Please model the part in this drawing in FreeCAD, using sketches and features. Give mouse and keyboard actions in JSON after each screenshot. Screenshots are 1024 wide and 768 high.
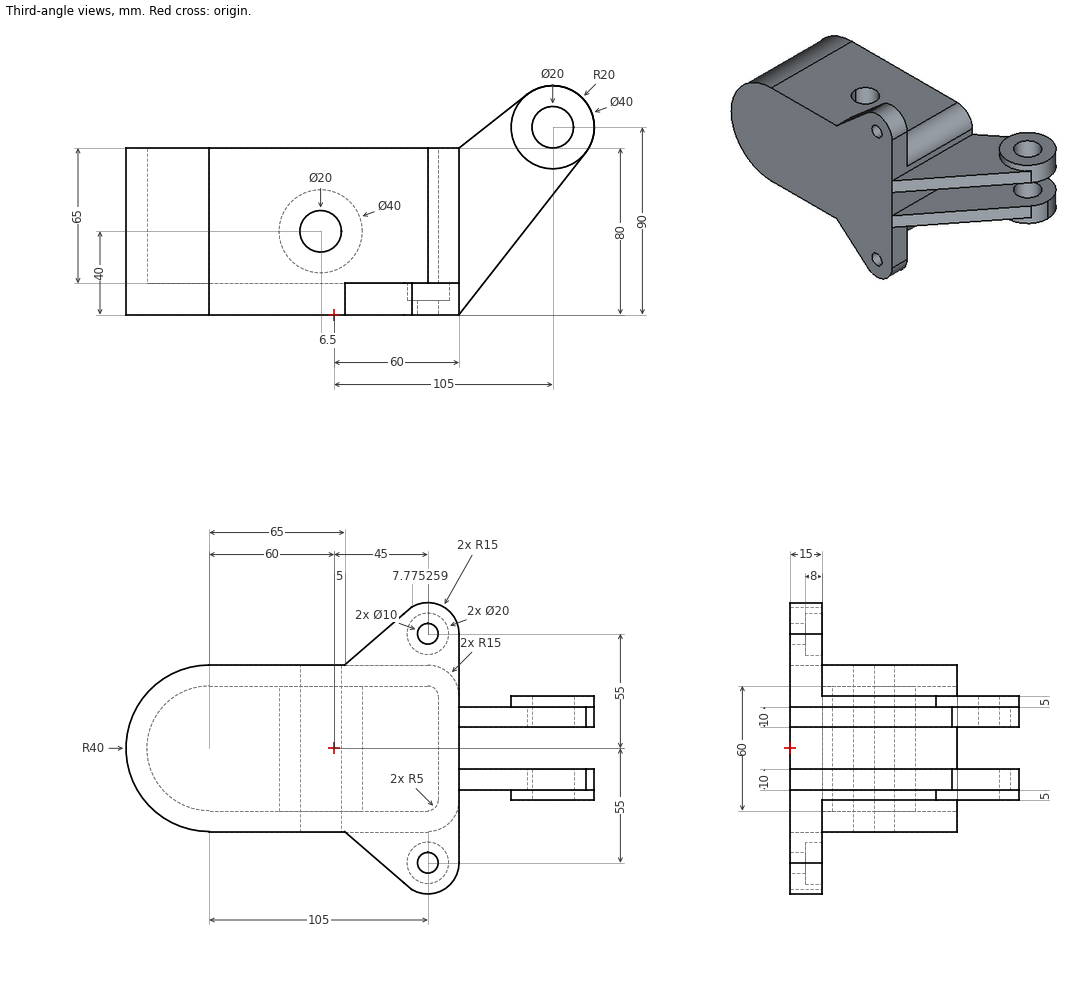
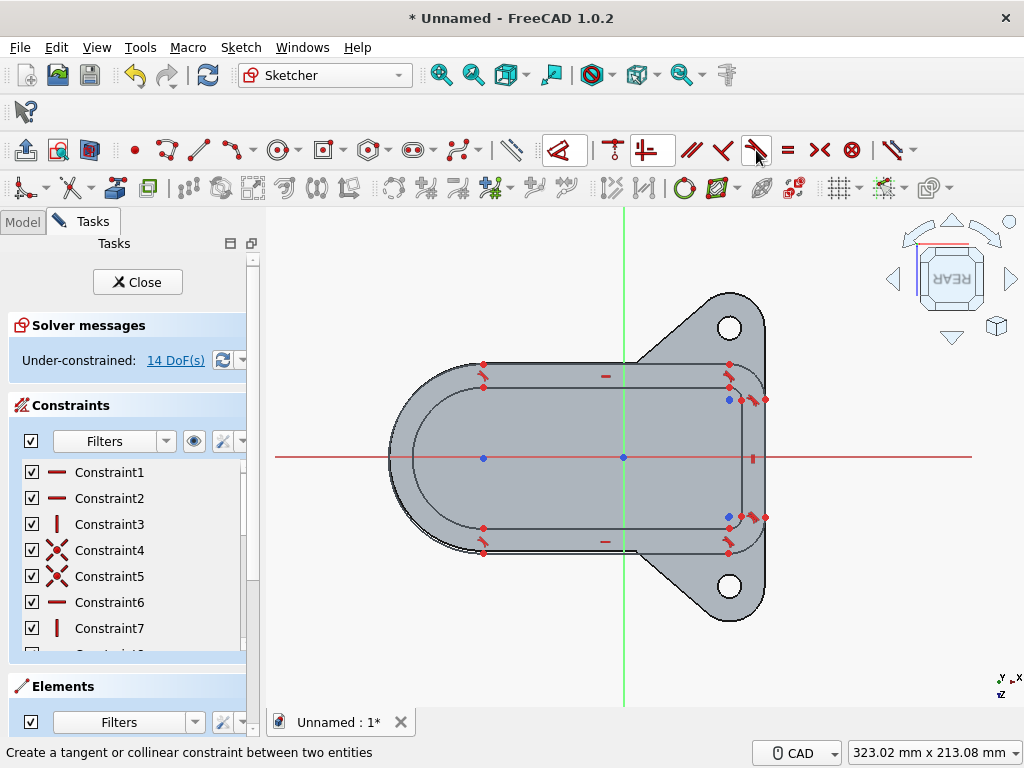
{"action": "left_click", "coordinate": [761, 384]}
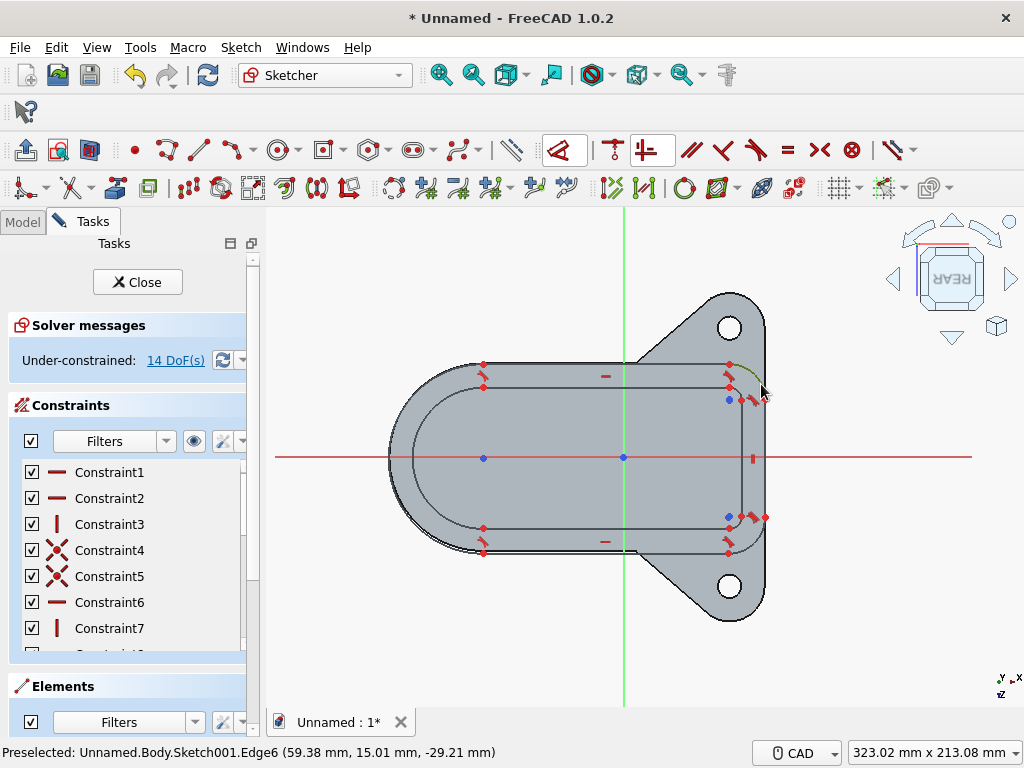
{"action": "scroll", "coordinate": [738, 391], "scroll_direction": "up", "scroll_amount": 2}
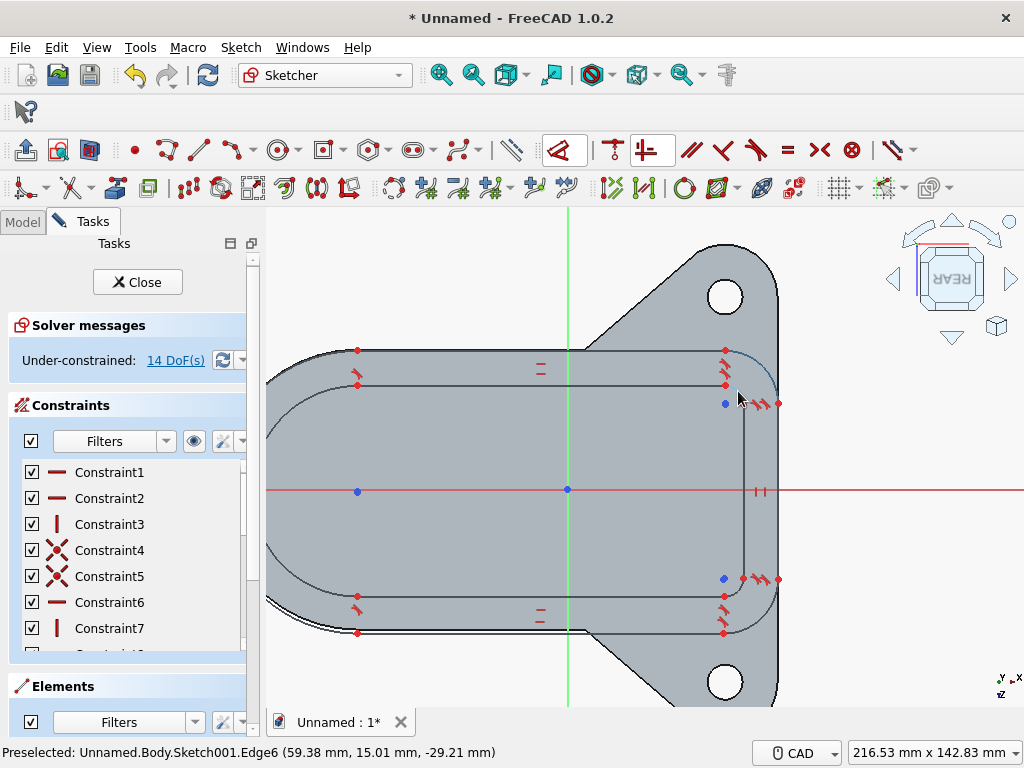
{"action": "left_click", "coordinate": [738, 391]}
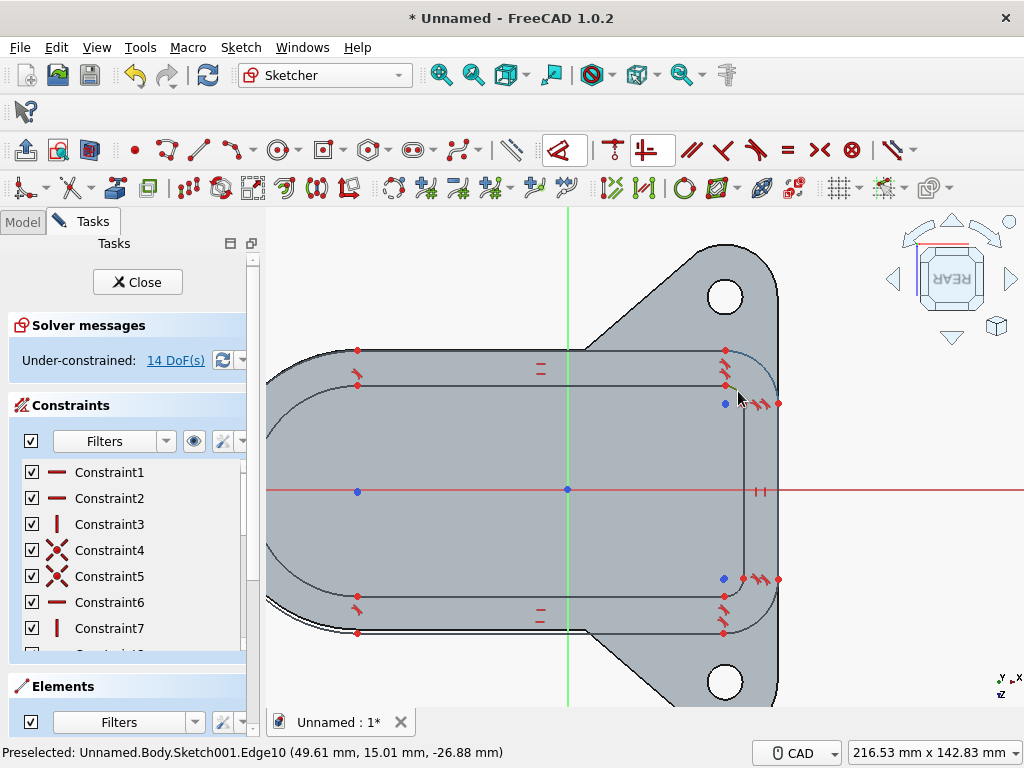
{"action": "left_click", "coordinate": [614, 150]}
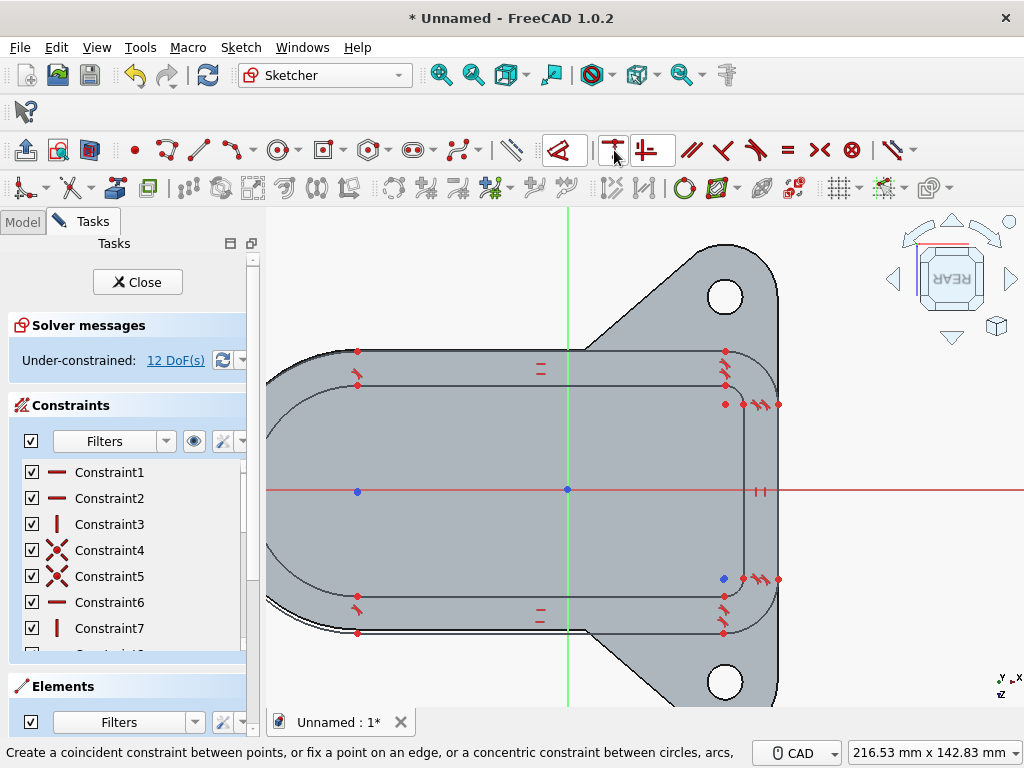
{"action": "left_click", "coordinate": [748, 628]}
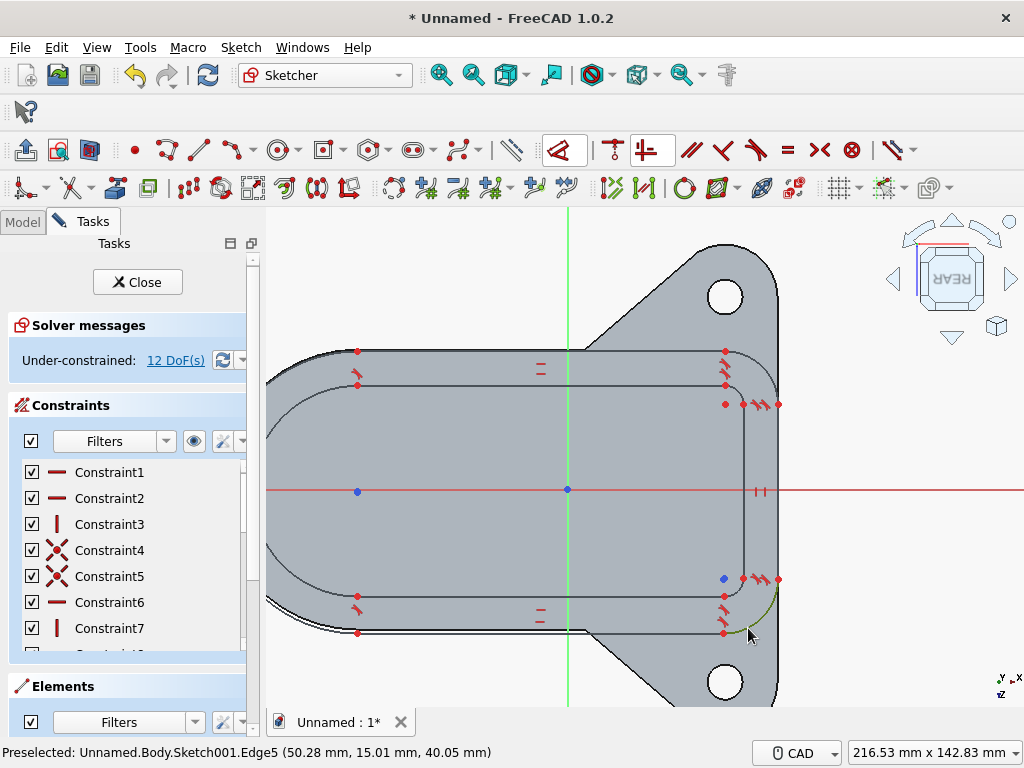
{"action": "left_click", "coordinate": [738, 591]}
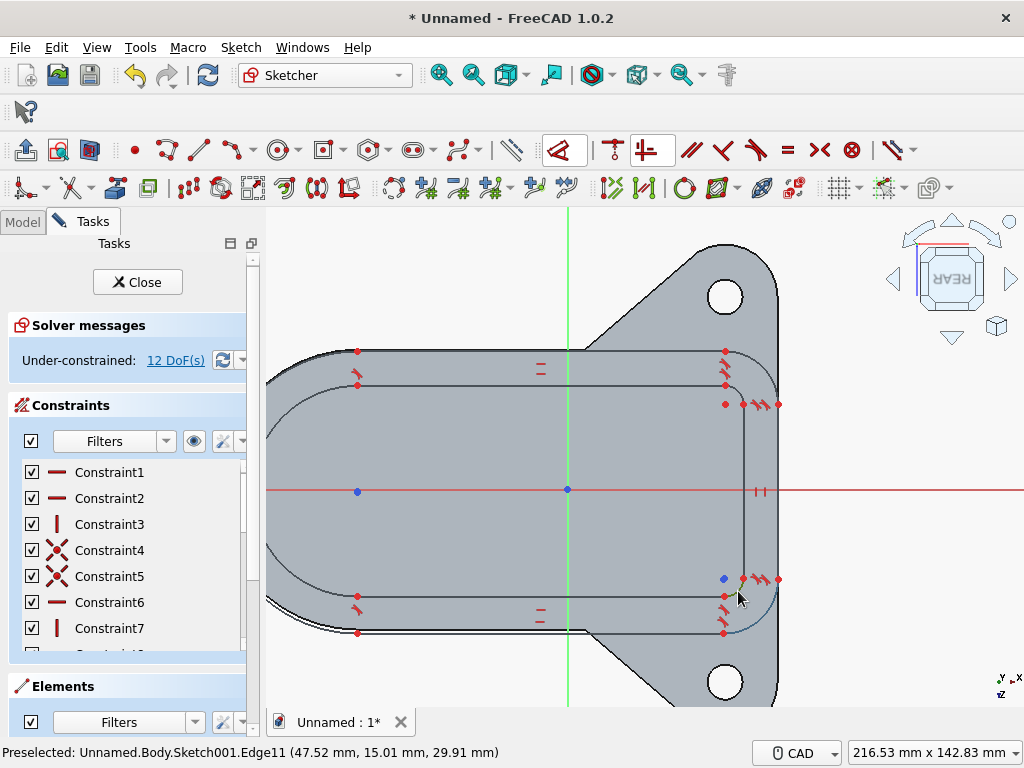
{"action": "left_click", "coordinate": [614, 150]}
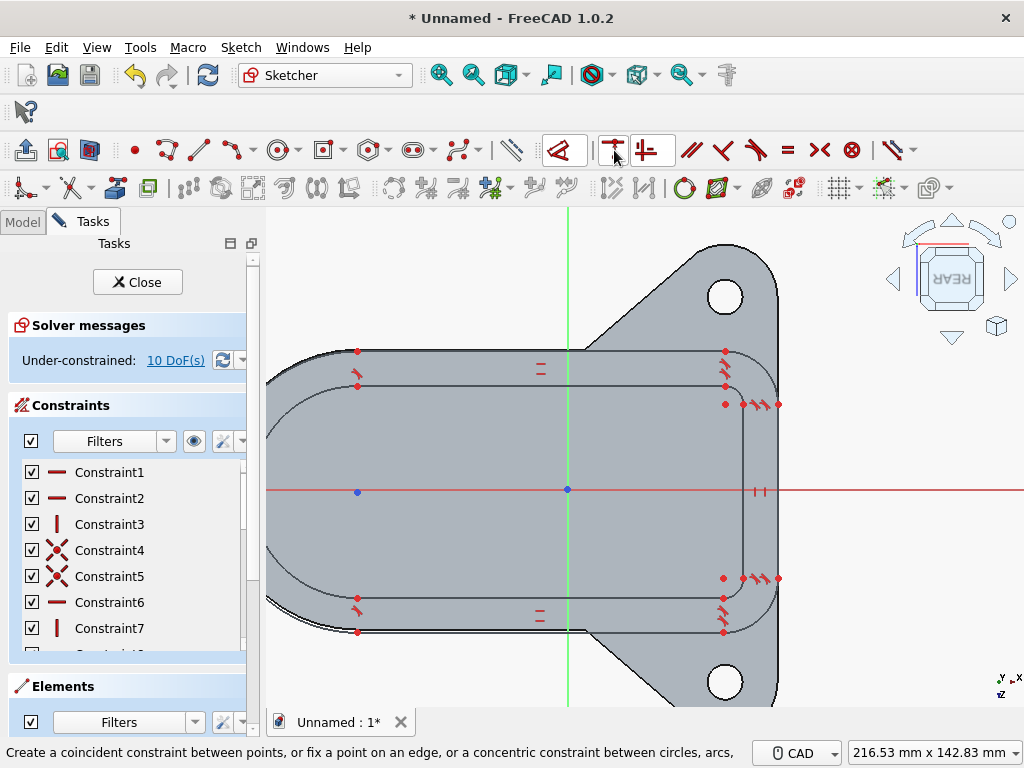
{"action": "left_click", "coordinate": [748, 627]}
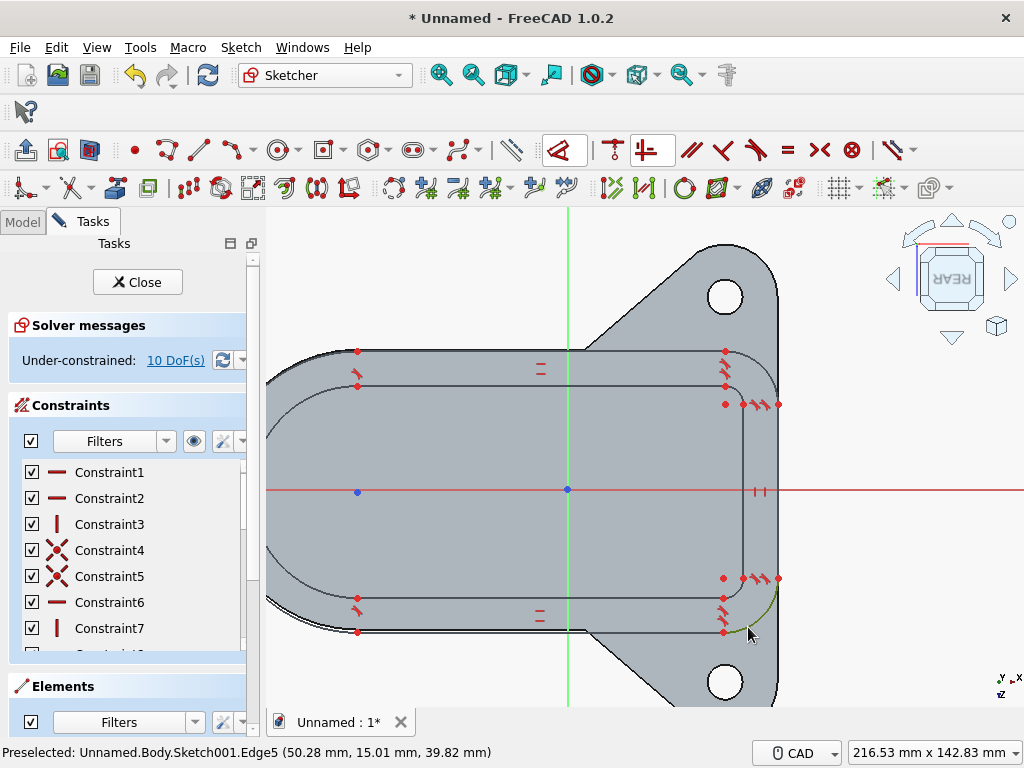
{"action": "left_click", "coordinate": [772, 380]}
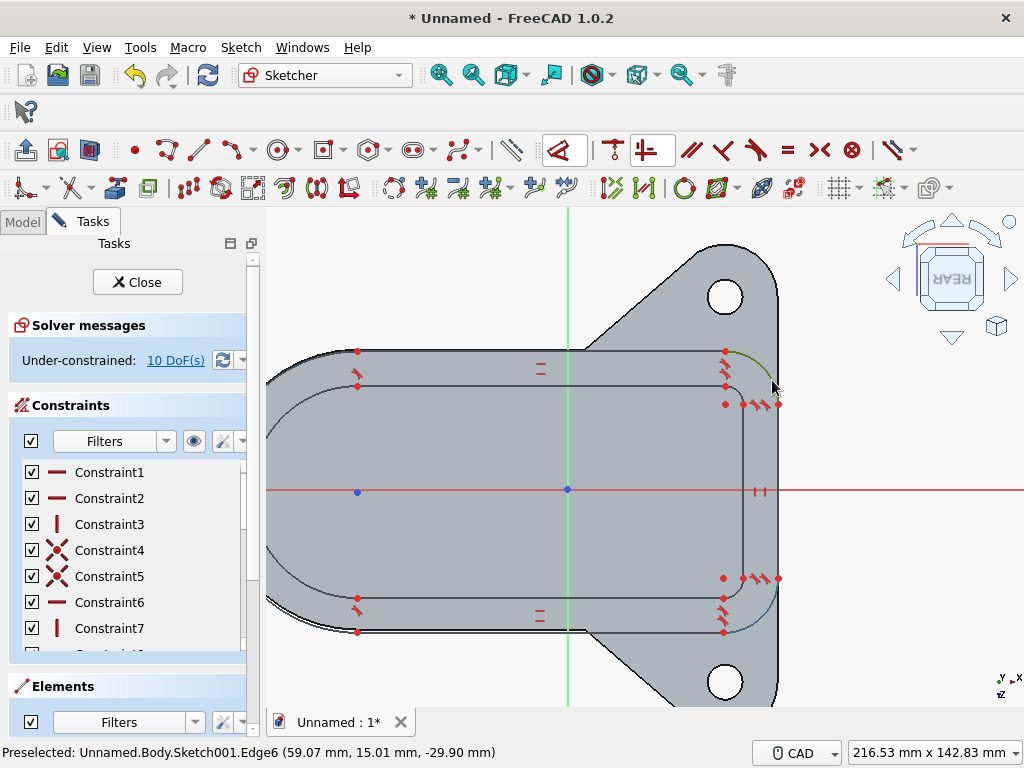
{"action": "left_click", "coordinate": [788, 150]}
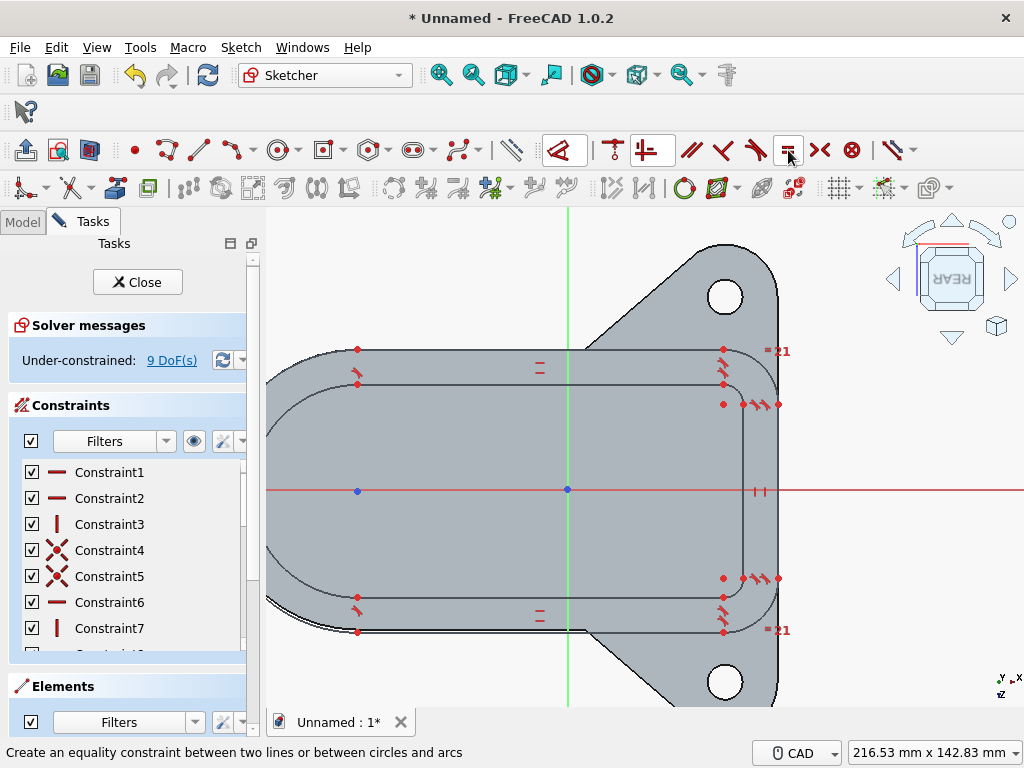
{"action": "left_click", "coordinate": [358, 491]}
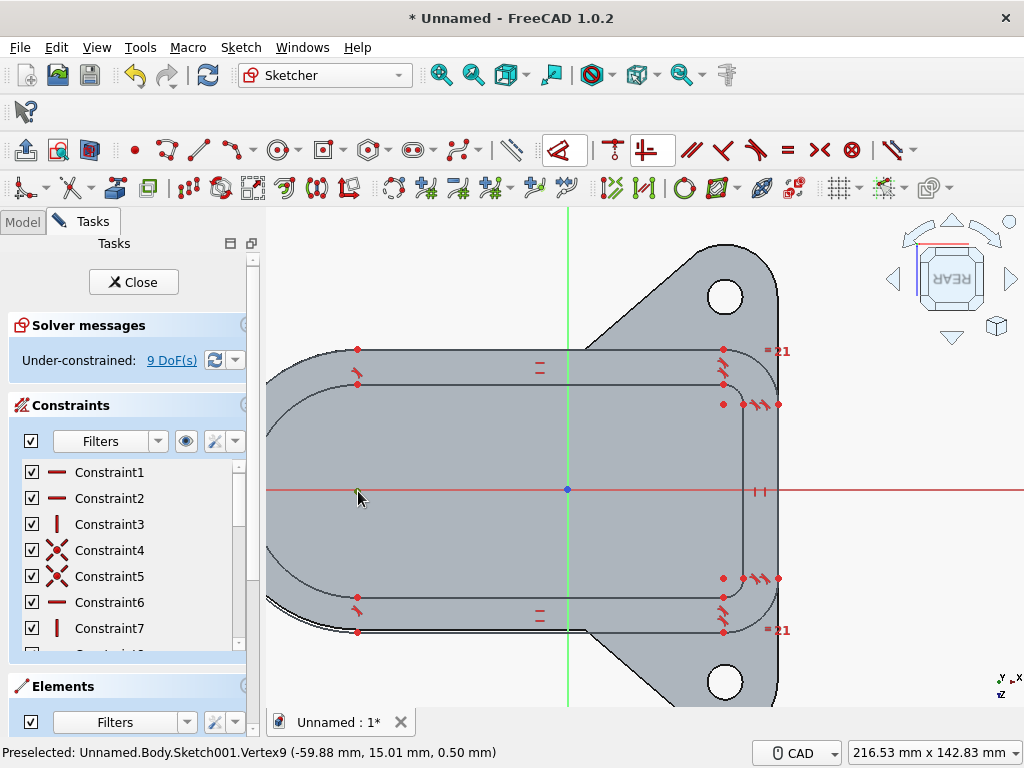
{"action": "left_click", "coordinate": [334, 490]}